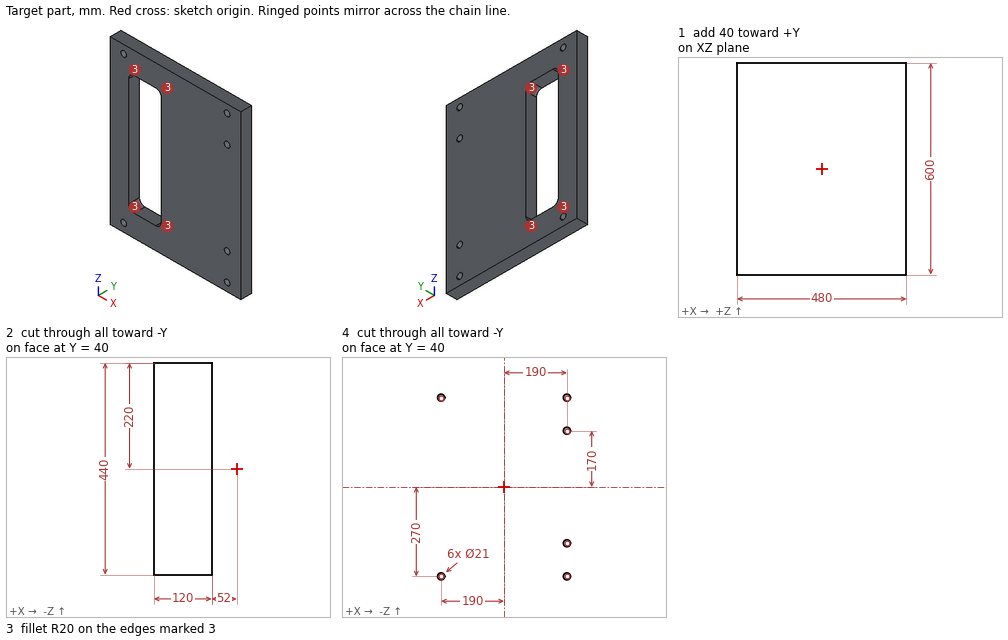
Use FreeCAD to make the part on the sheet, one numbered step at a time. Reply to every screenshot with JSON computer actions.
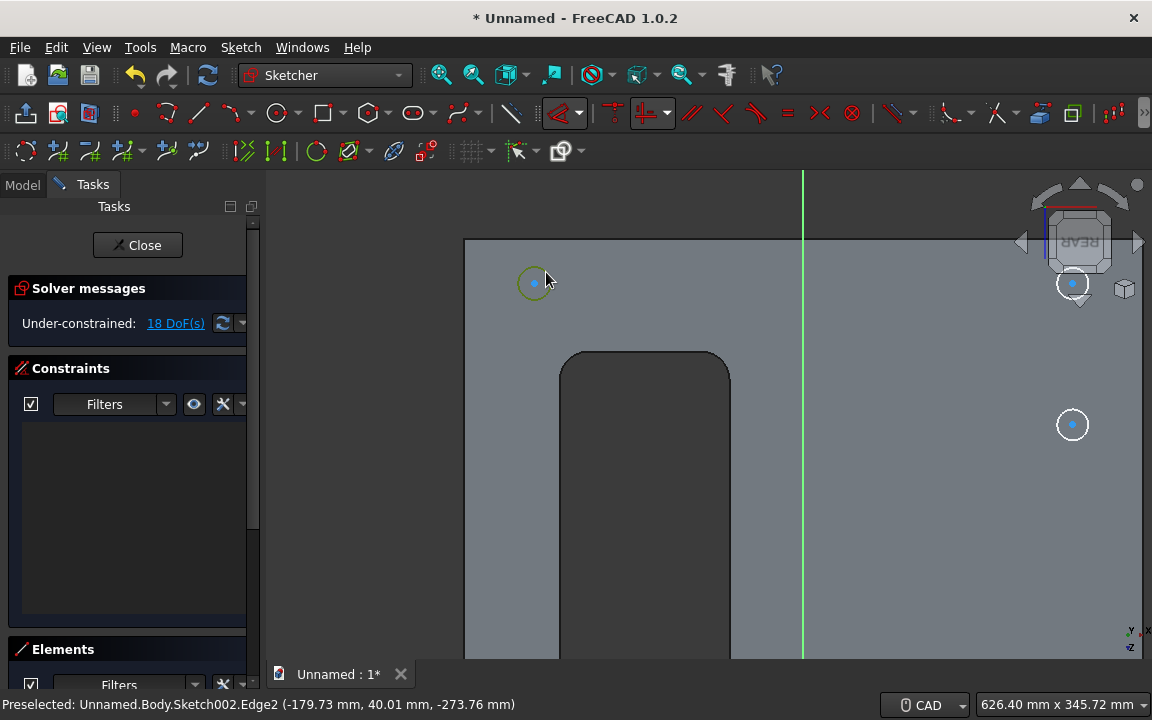
{"action": "scroll", "coordinate": [546, 270], "scroll_direction": "down", "scroll_amount": 5}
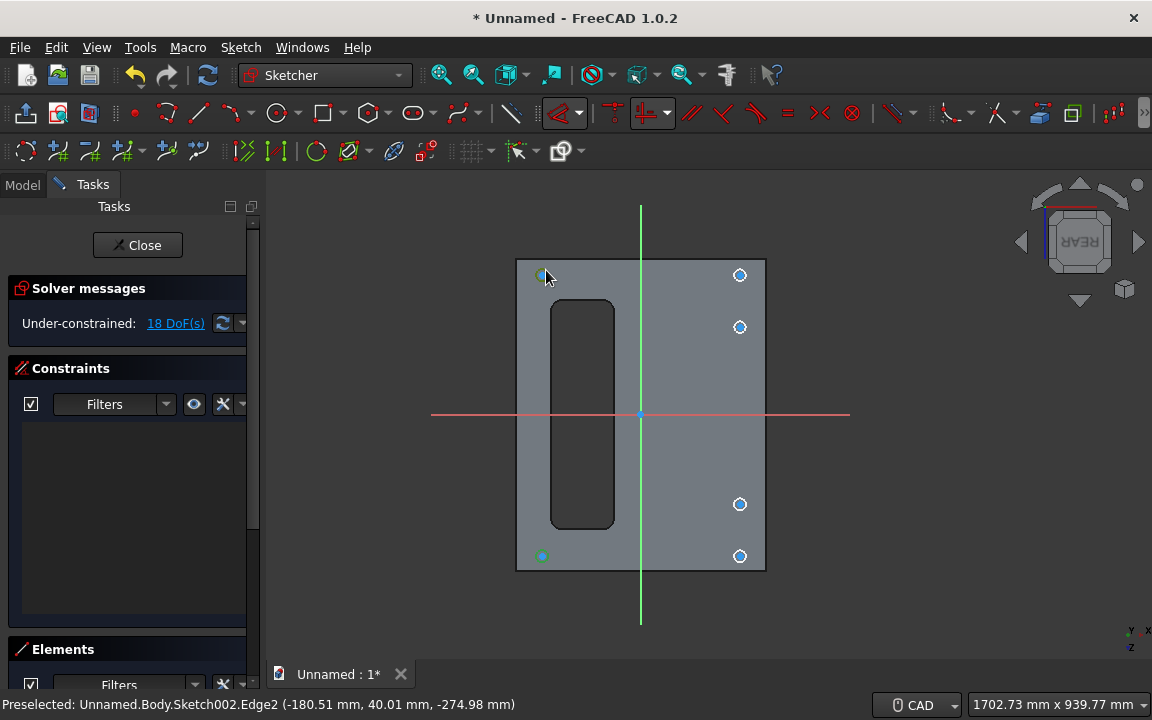
{"action": "scroll", "coordinate": [744, 271], "scroll_direction": "up", "scroll_amount": 5}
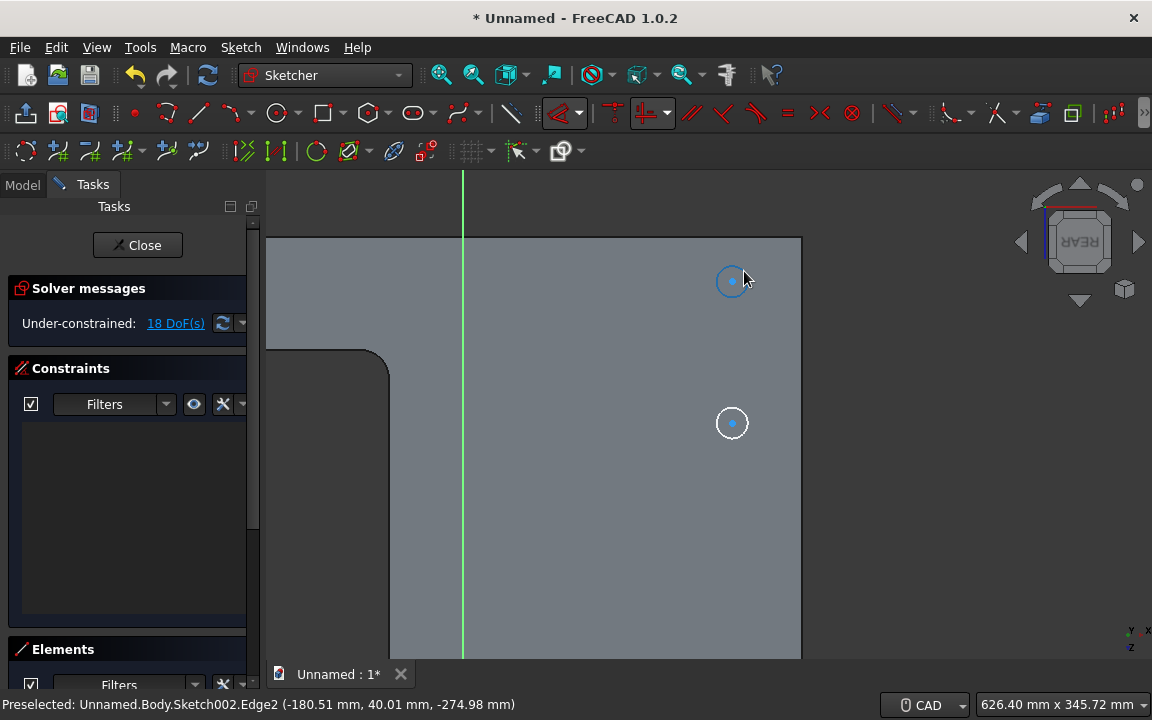
{"action": "left_click", "coordinate": [743, 271]}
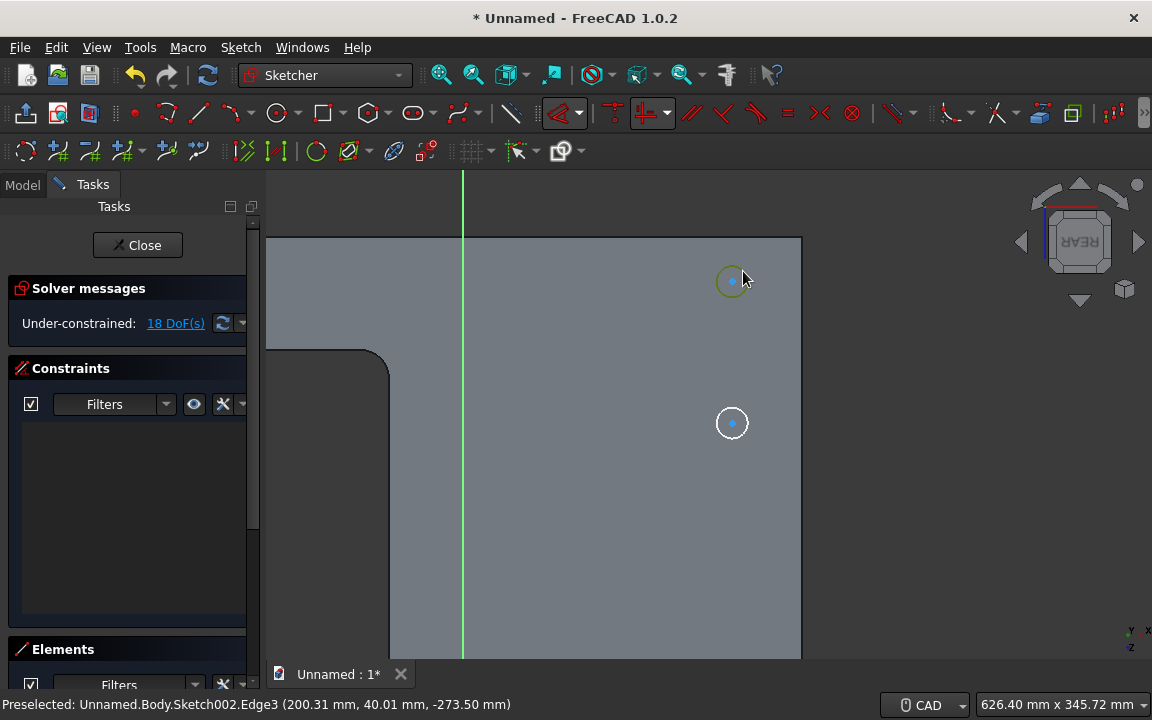
{"action": "scroll", "coordinate": [744, 271], "scroll_direction": "down", "scroll_amount": 5}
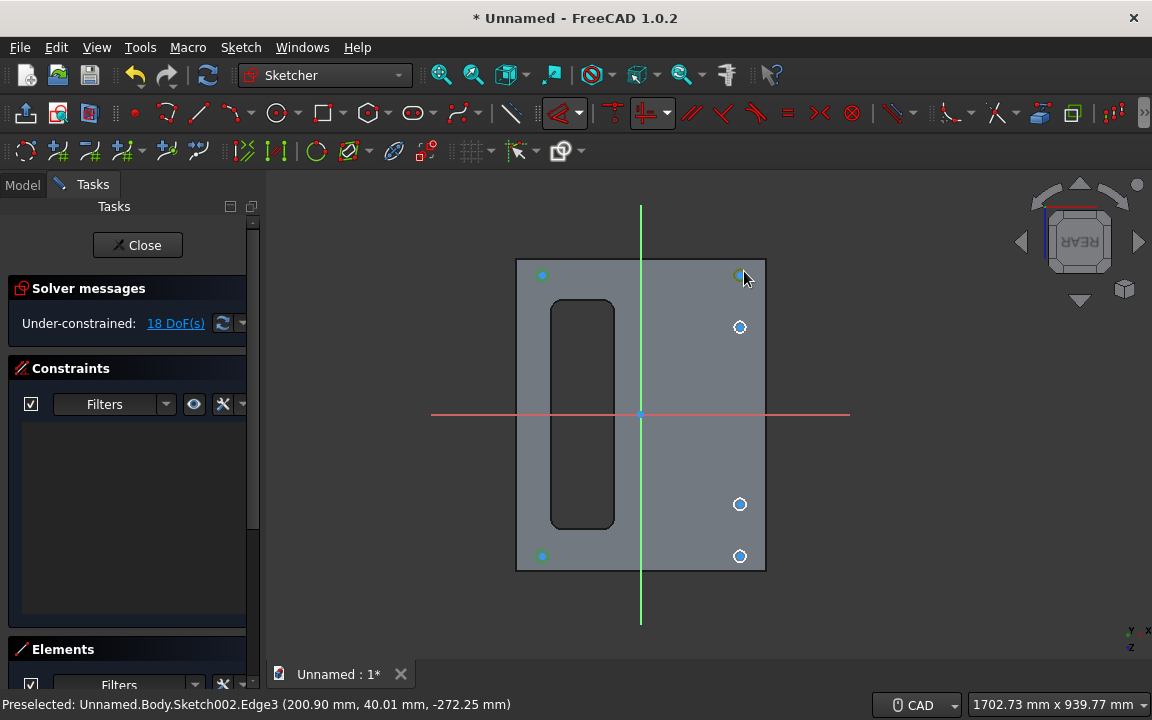
{"action": "scroll", "coordinate": [744, 552], "scroll_direction": "up", "scroll_amount": 5}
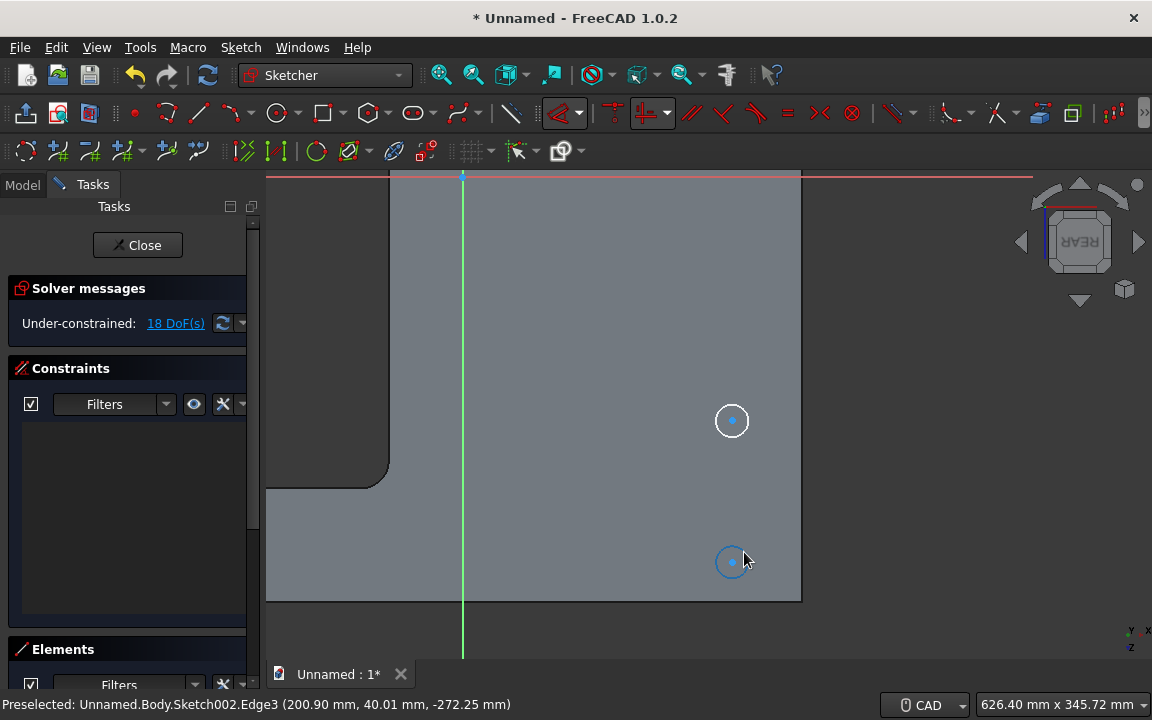
{"action": "left_click", "coordinate": [743, 551]}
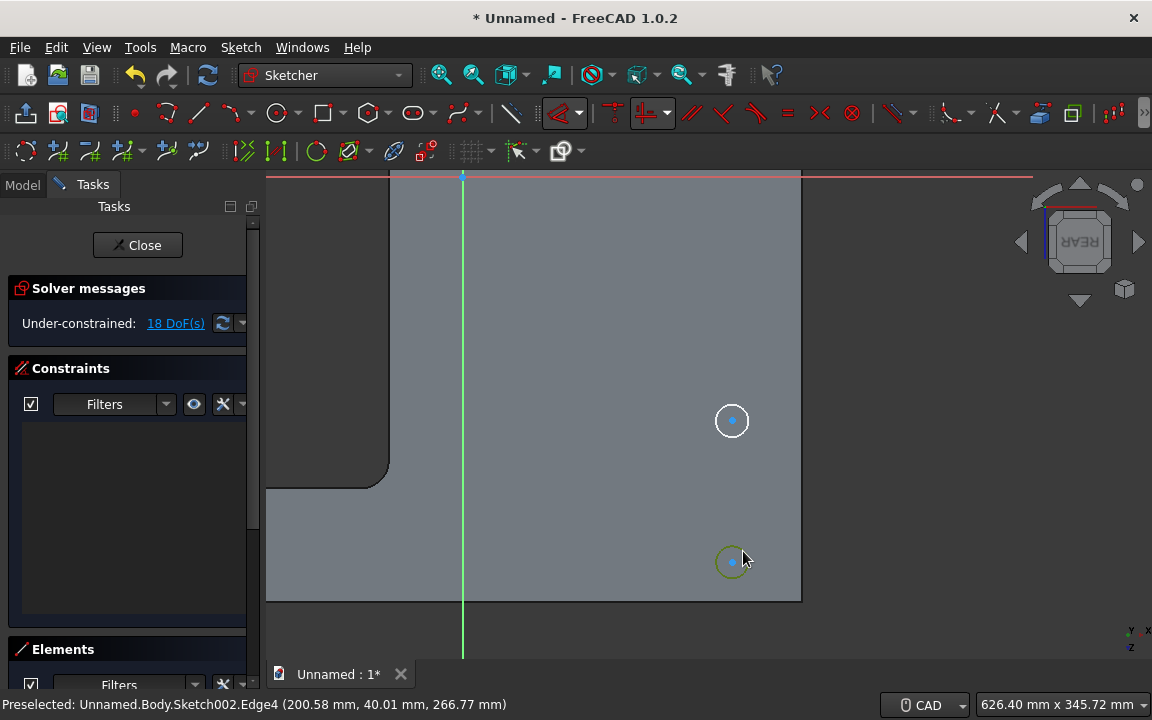
{"action": "scroll", "coordinate": [744, 553], "scroll_direction": "down", "scroll_amount": 5}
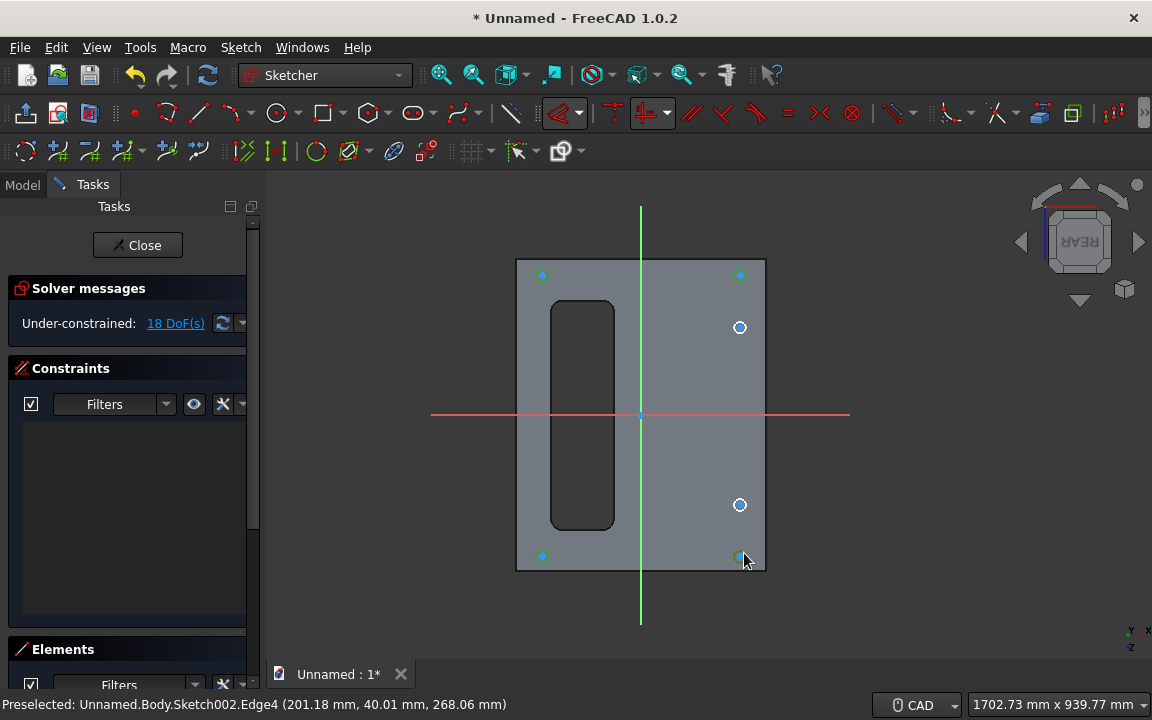
{"action": "scroll", "coordinate": [744, 324], "scroll_direction": "up", "scroll_amount": 5}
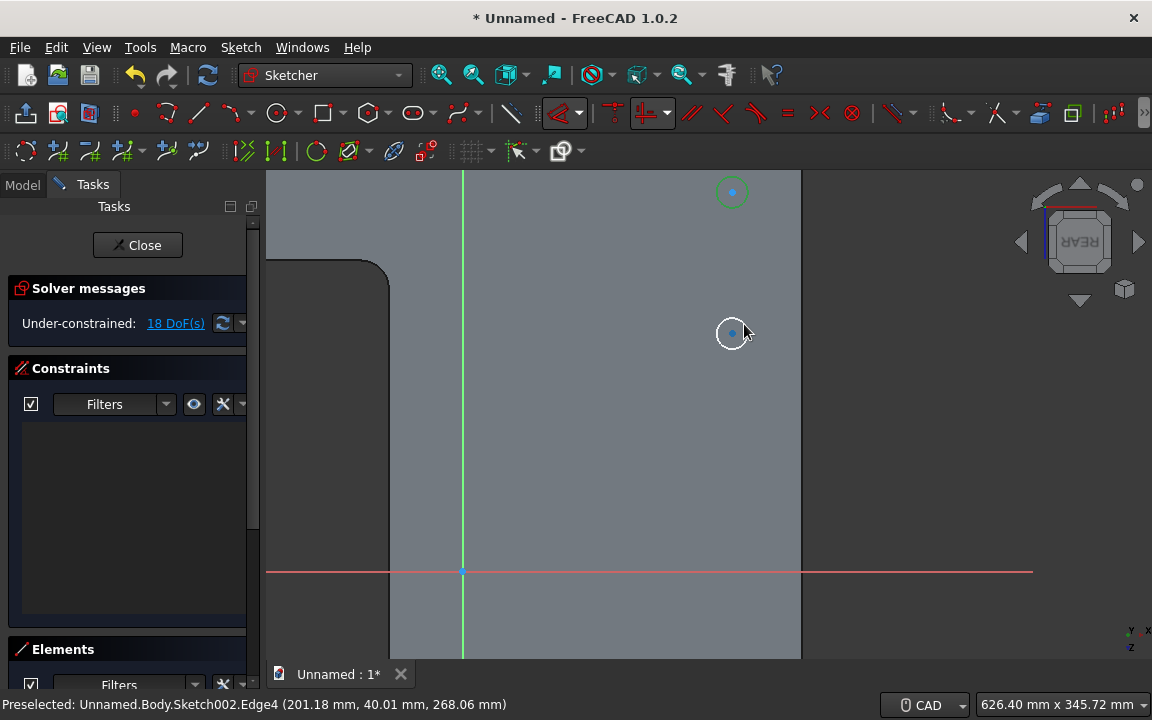
{"action": "left_click", "coordinate": [743, 323]}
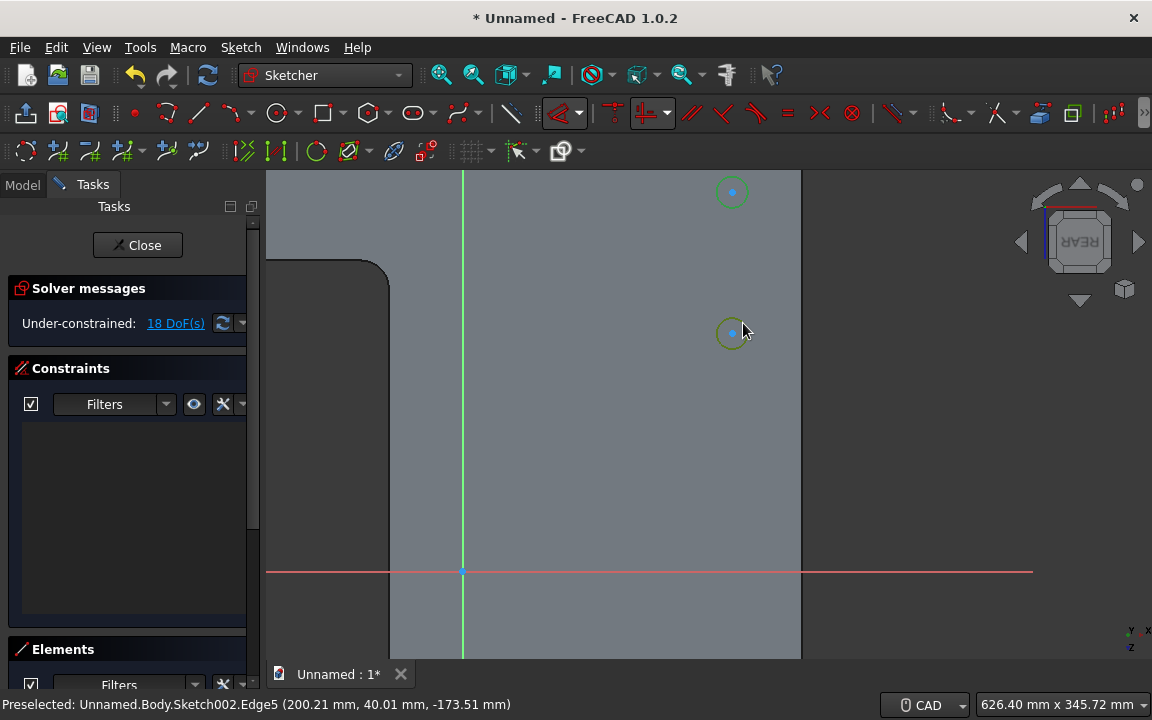
{"action": "scroll", "coordinate": [744, 323], "scroll_direction": "down", "scroll_amount": 5}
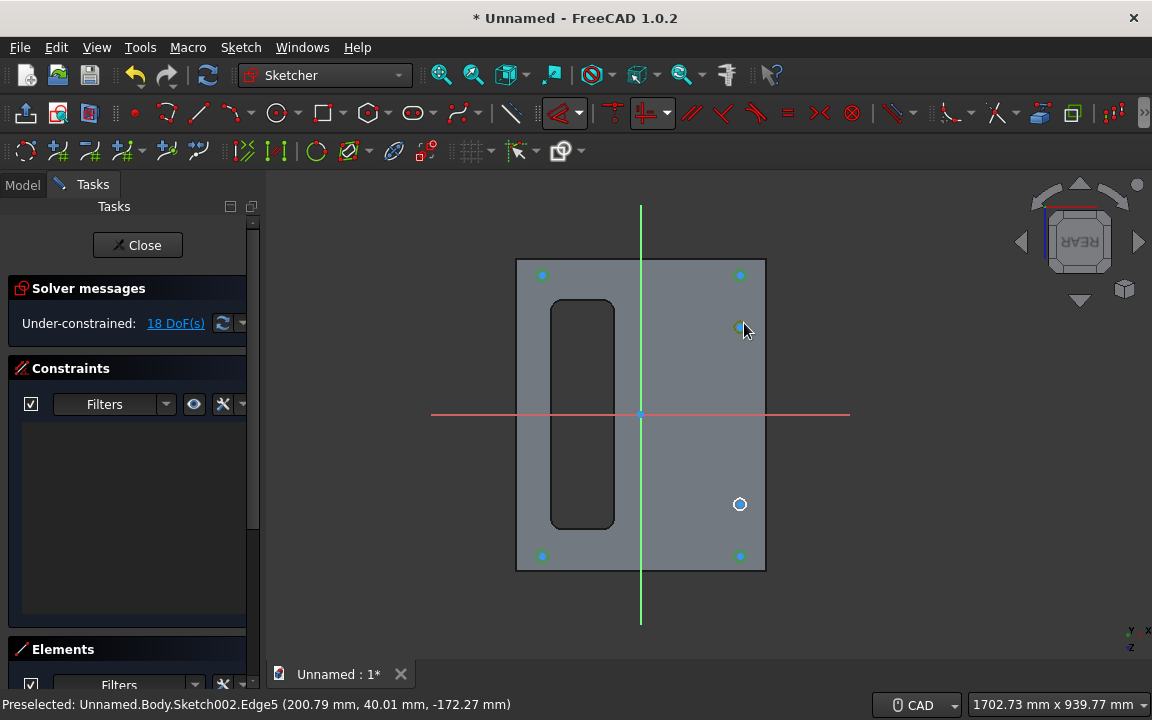
{"action": "scroll", "coordinate": [744, 500], "scroll_direction": "up", "scroll_amount": 5}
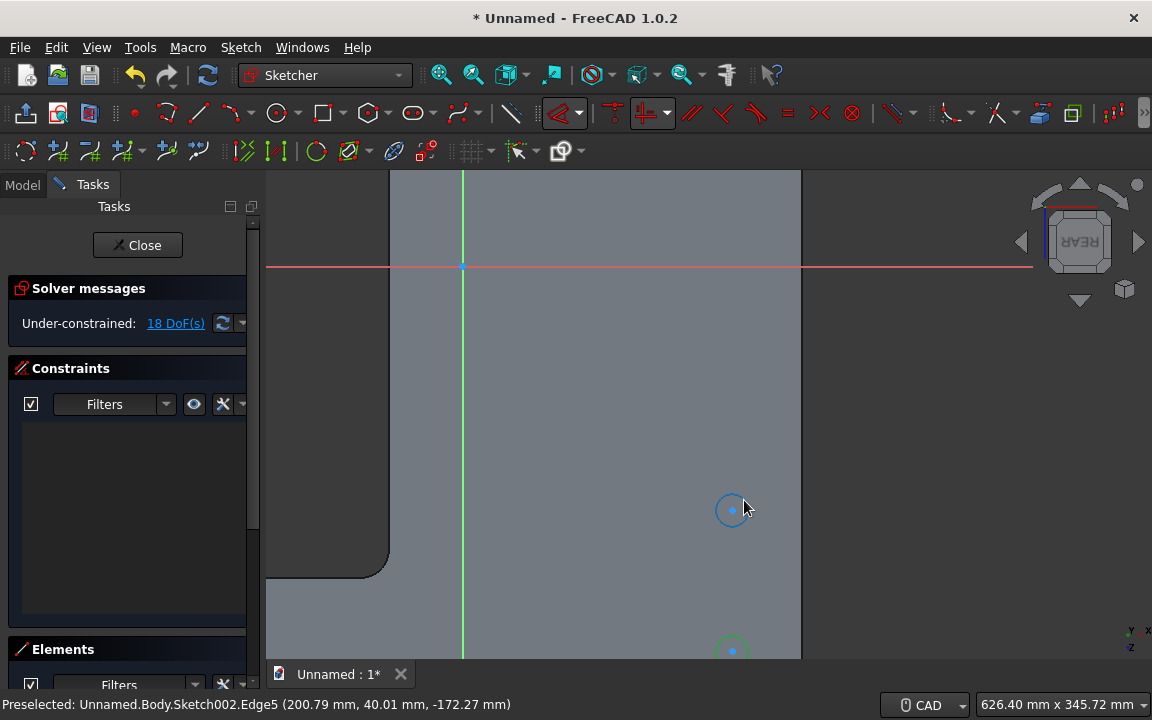
{"action": "left_click", "coordinate": [744, 499]}